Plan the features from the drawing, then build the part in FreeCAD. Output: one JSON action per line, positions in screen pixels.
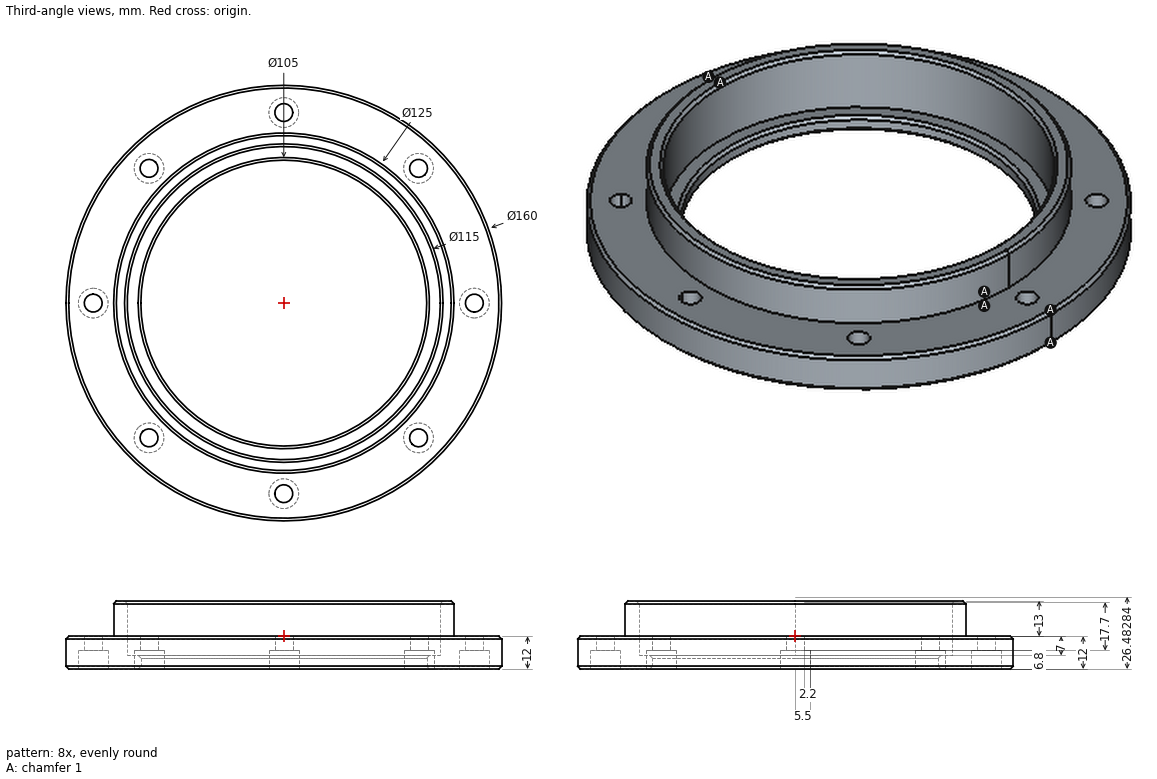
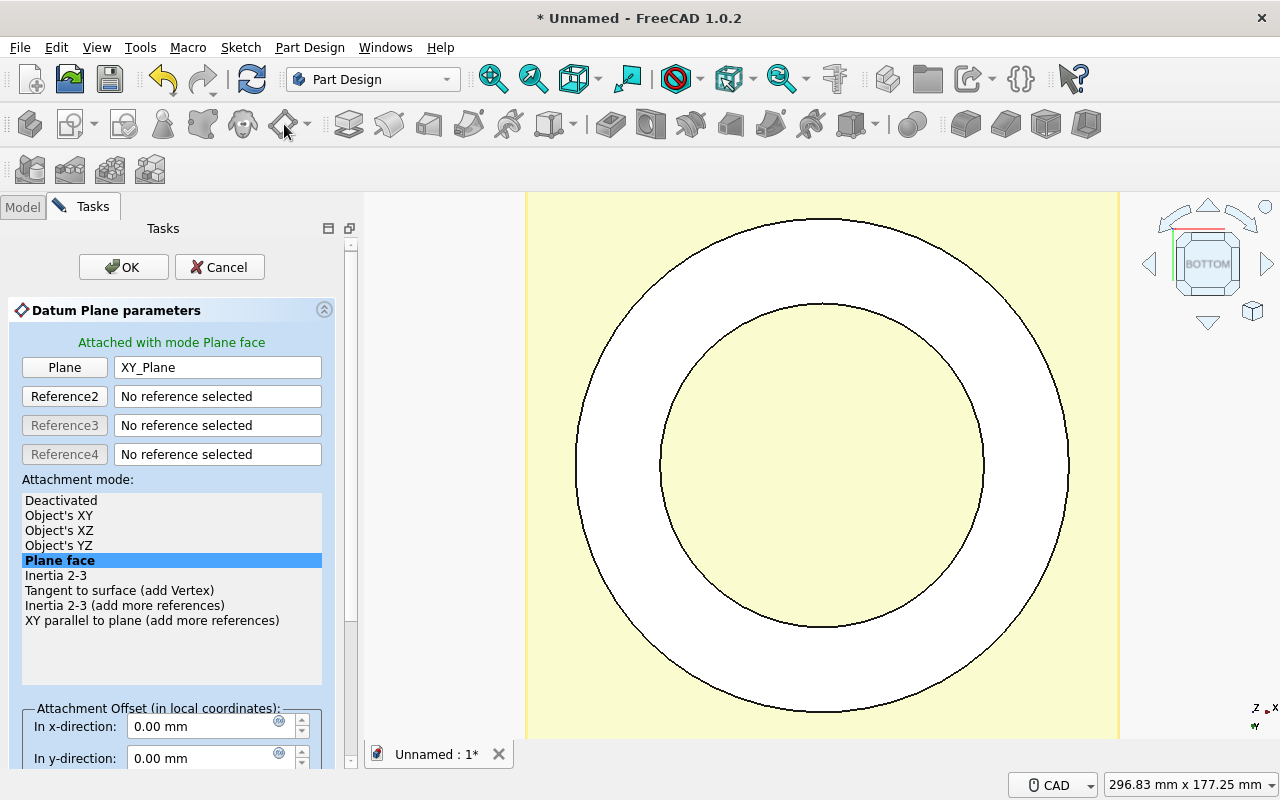
{"action": "scroll", "coordinate": [351, 503], "scroll_direction": "down", "scroll_amount": 2}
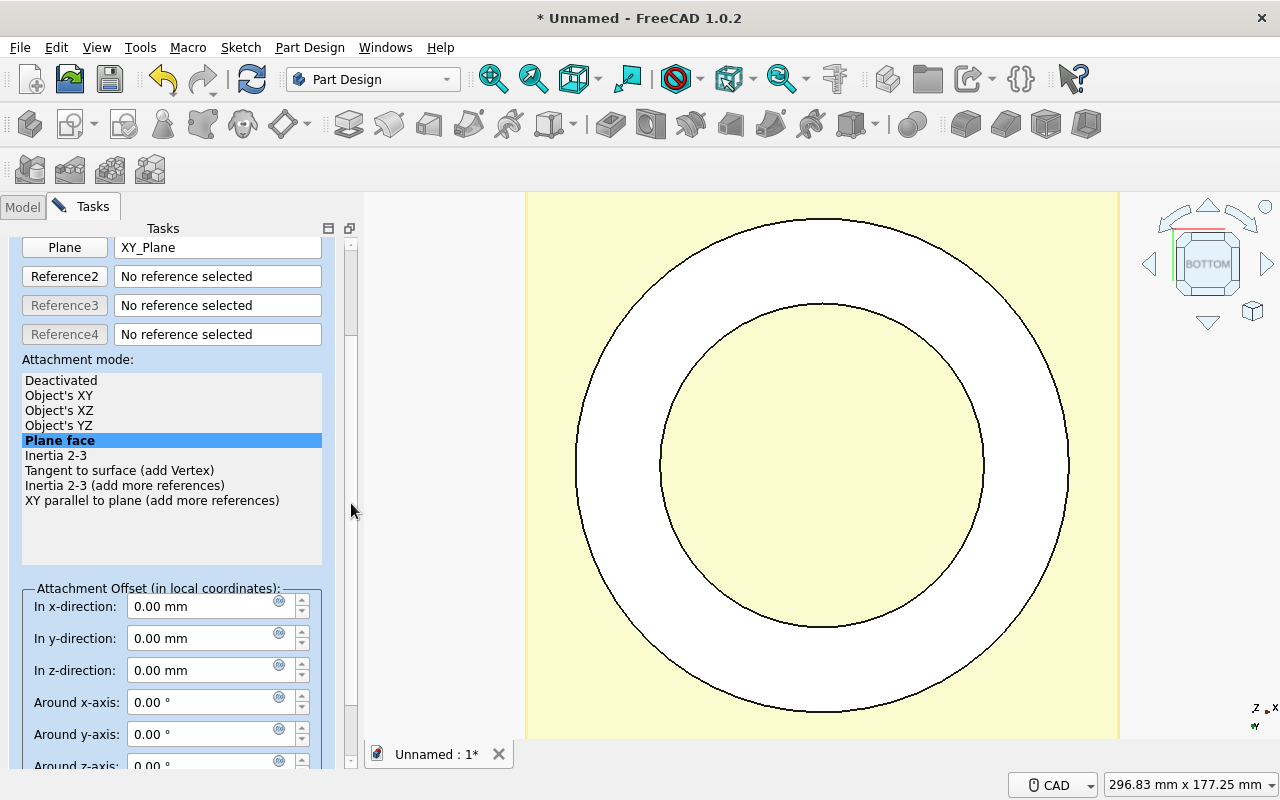
{"action": "triple_click", "coordinate": [210, 670]}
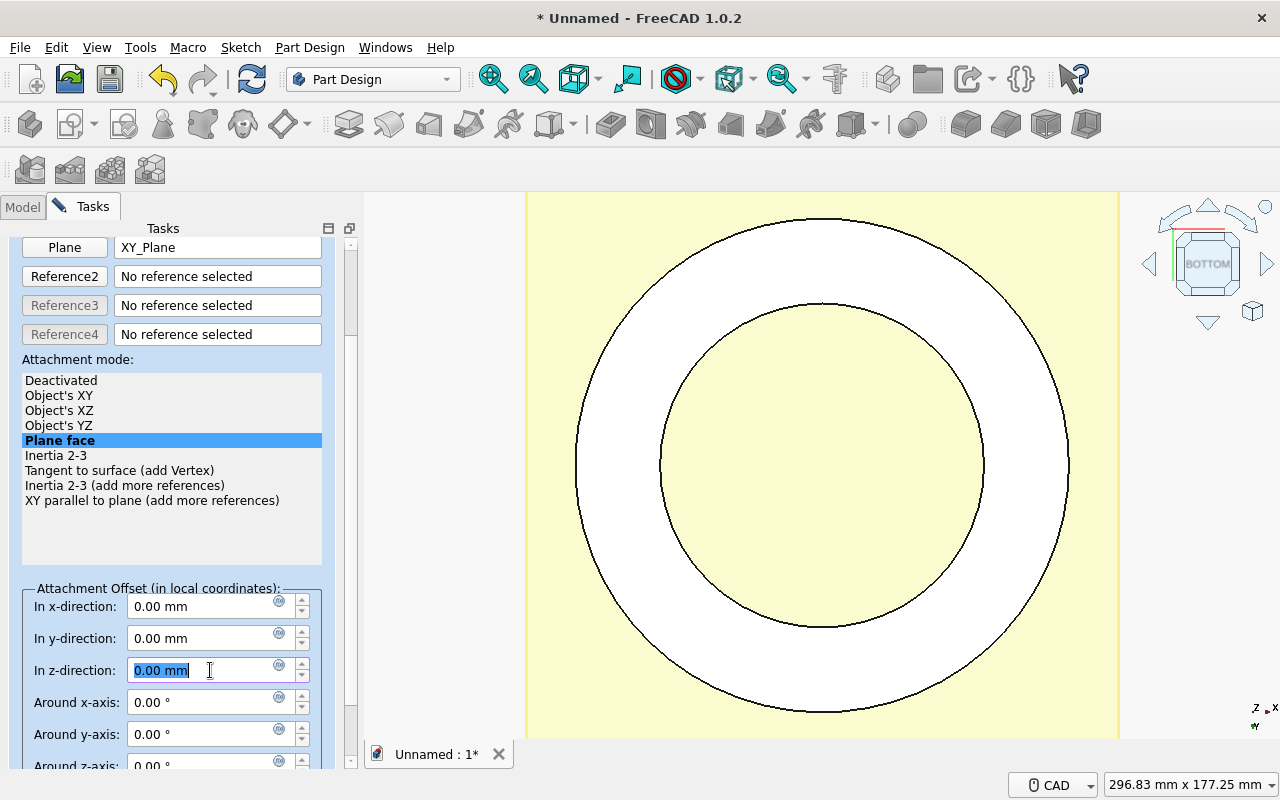
{"action": "type", "text": "-7"}
{"action": "key", "text": "Tab"}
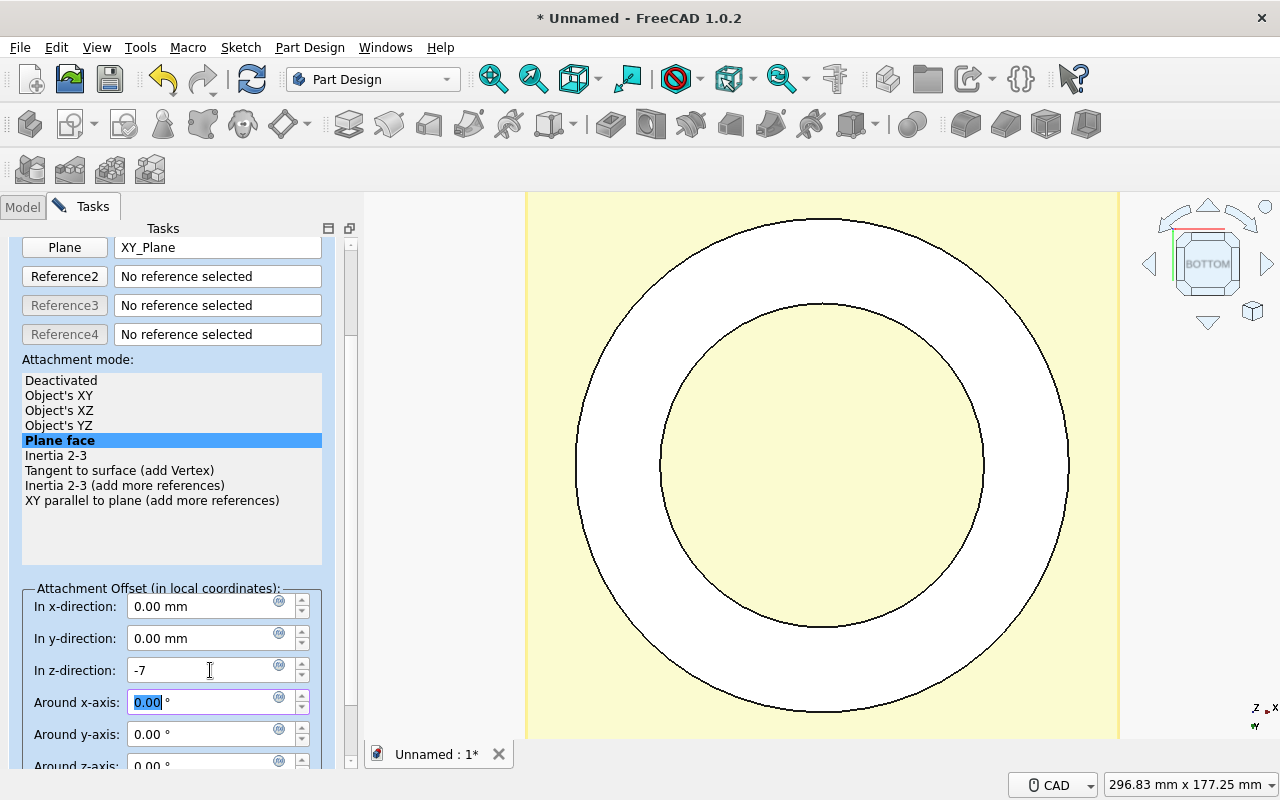
{"action": "scroll", "coordinate": [351, 503], "scroll_direction": "up", "scroll_amount": 3}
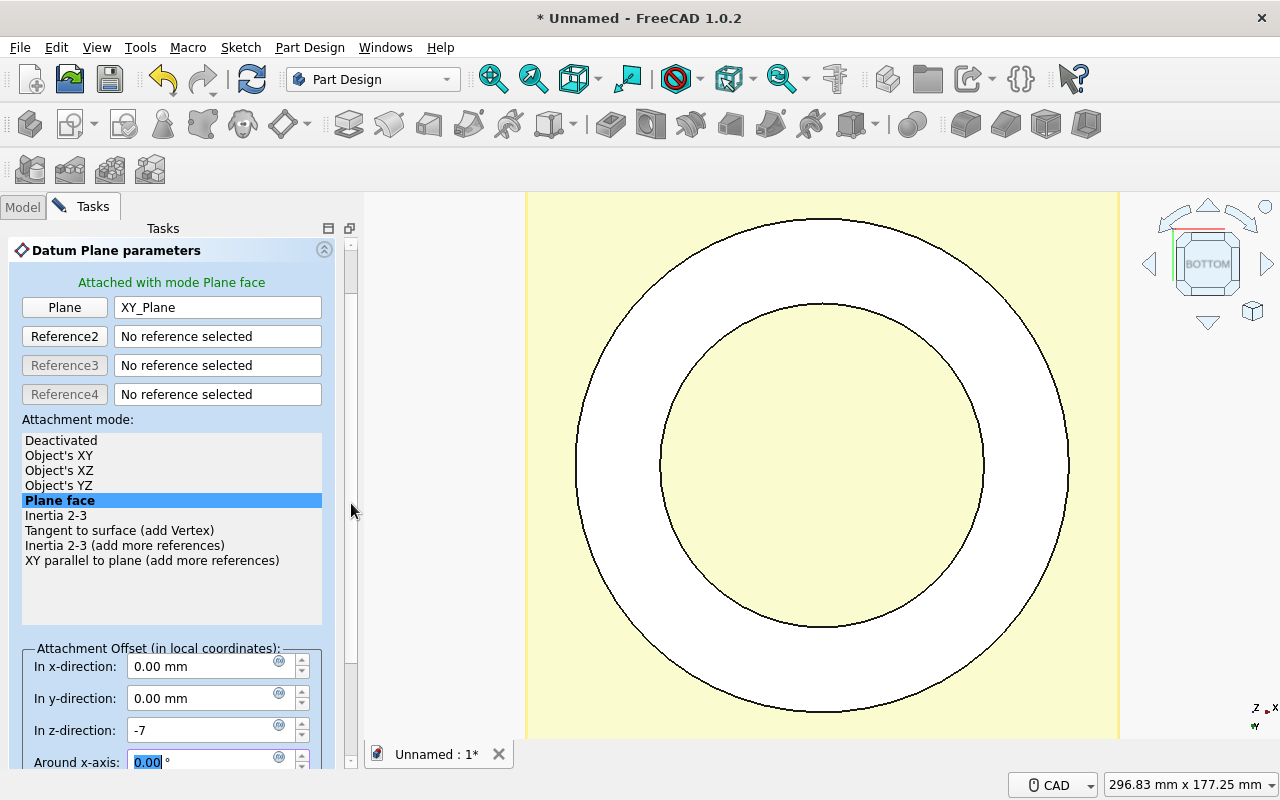
{"action": "left_click", "coordinate": [124, 267]}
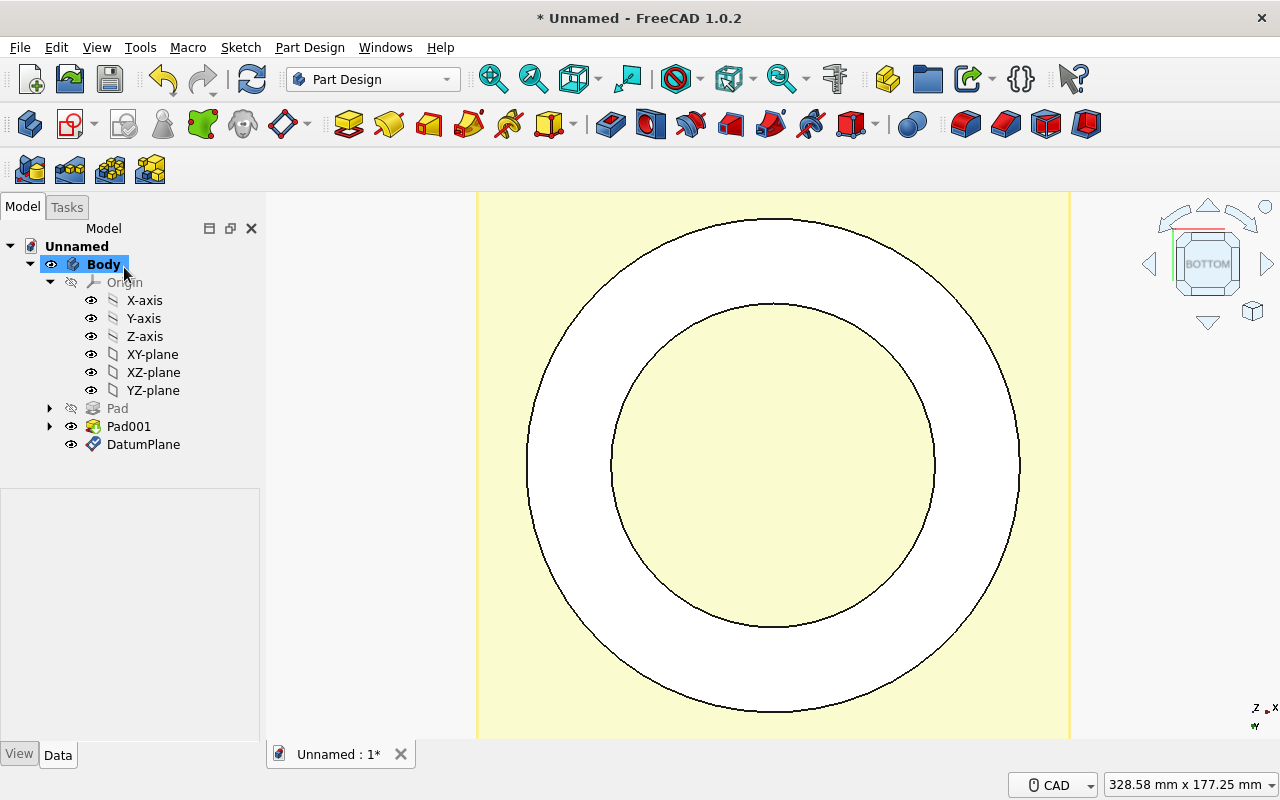
{"action": "left_click", "coordinate": [116, 444]}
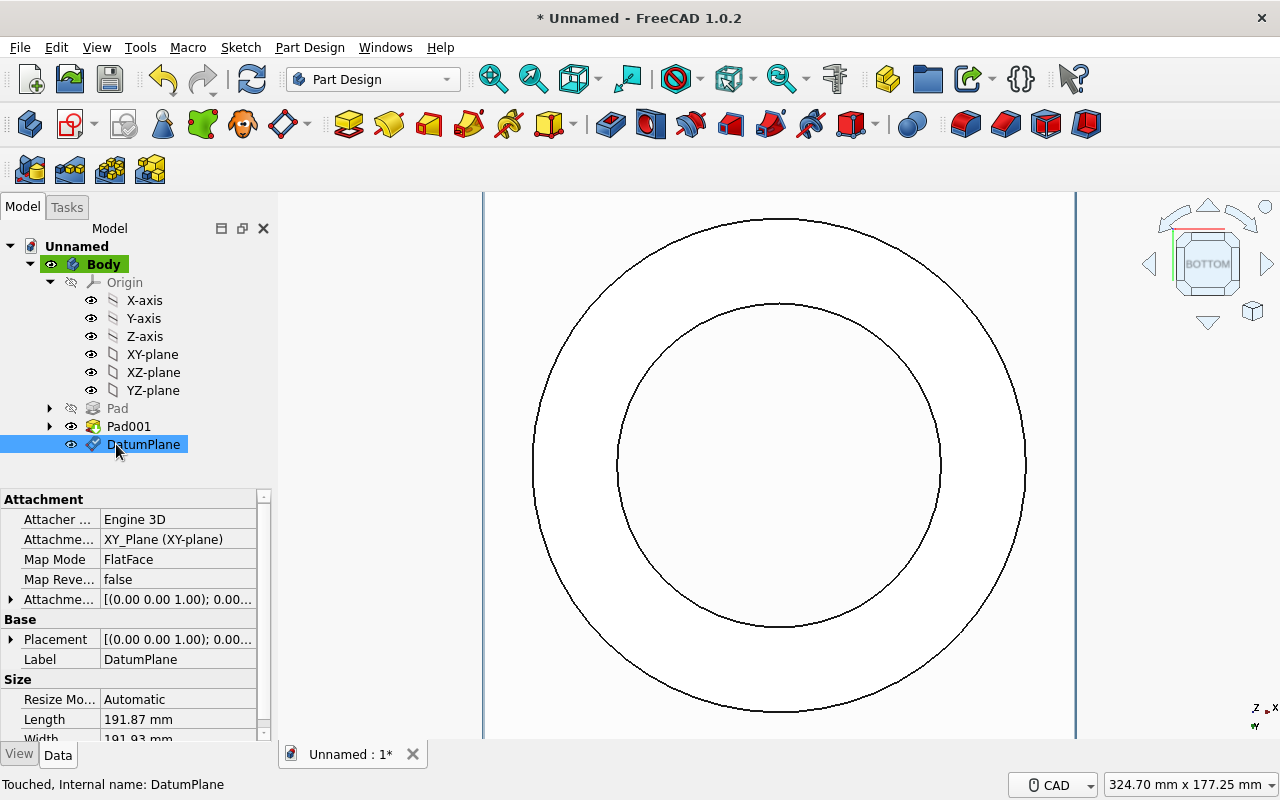
{"action": "left_click", "coordinate": [70, 124]}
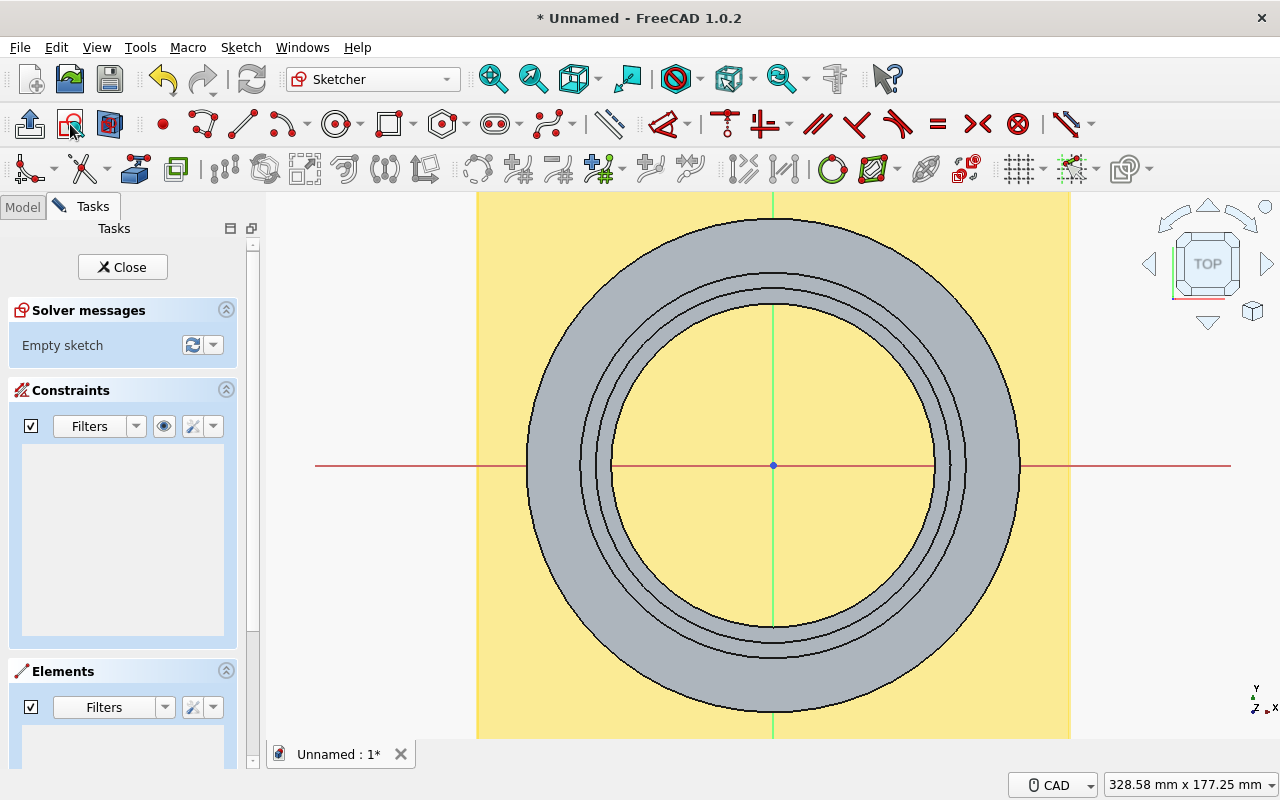
{"action": "left_click", "coordinate": [110, 124]}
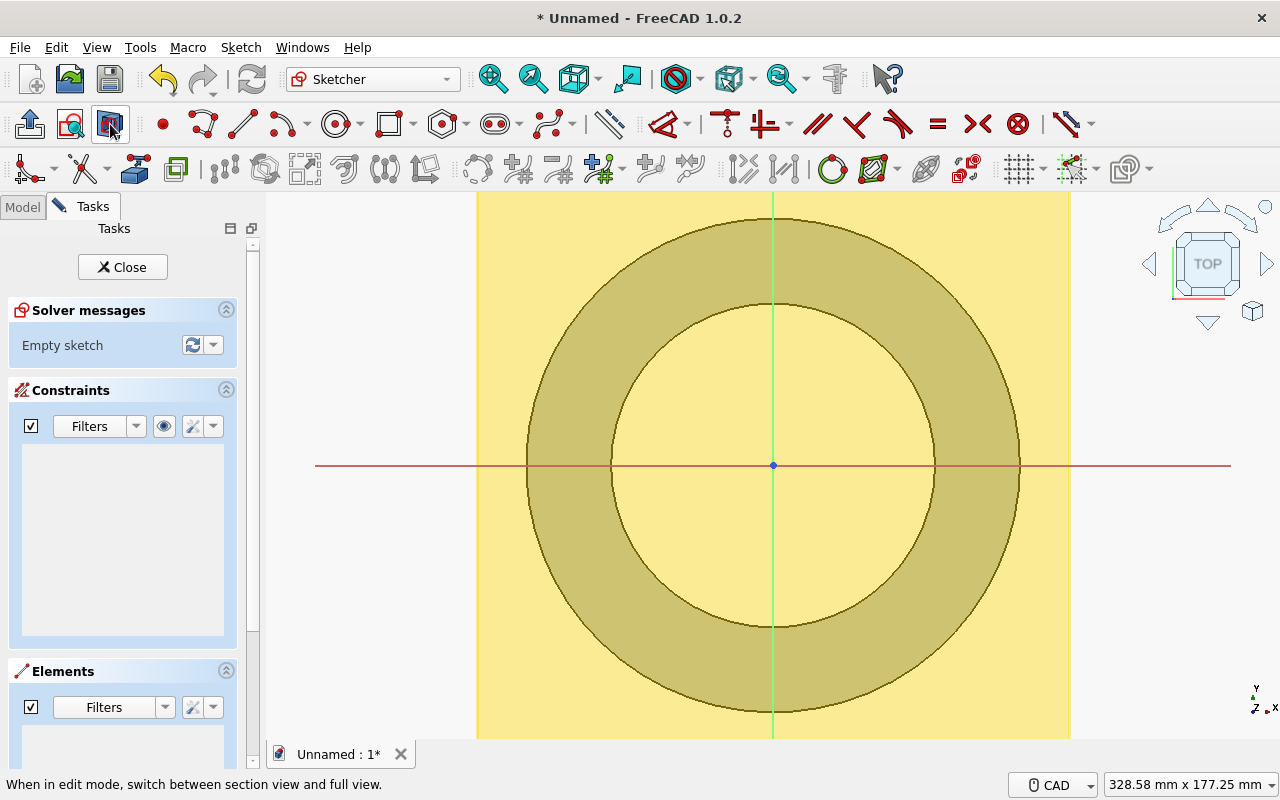
{"action": "left_click", "coordinate": [336, 124]}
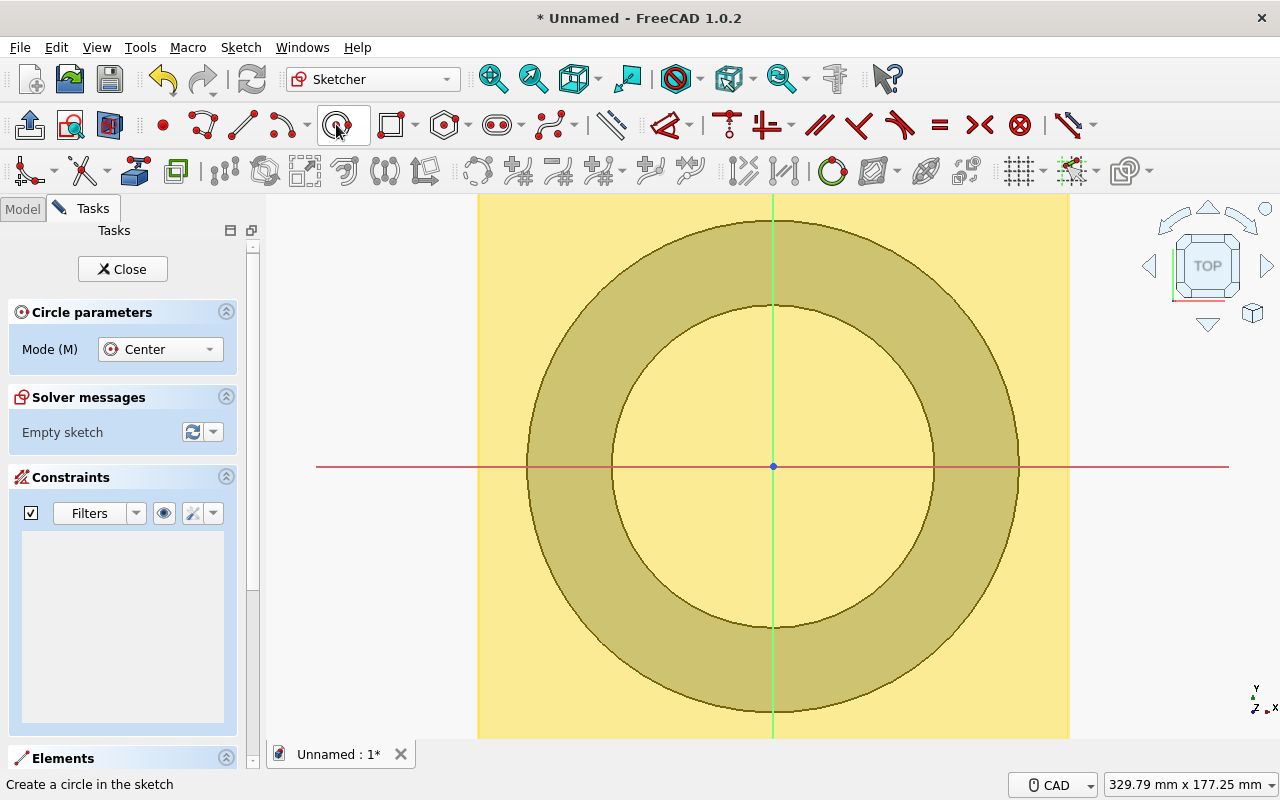
{"action": "left_click", "coordinate": [773, 466]}
{"action": "left_click", "coordinate": [898, 341]}
{"action": "key", "text": "Escape"}